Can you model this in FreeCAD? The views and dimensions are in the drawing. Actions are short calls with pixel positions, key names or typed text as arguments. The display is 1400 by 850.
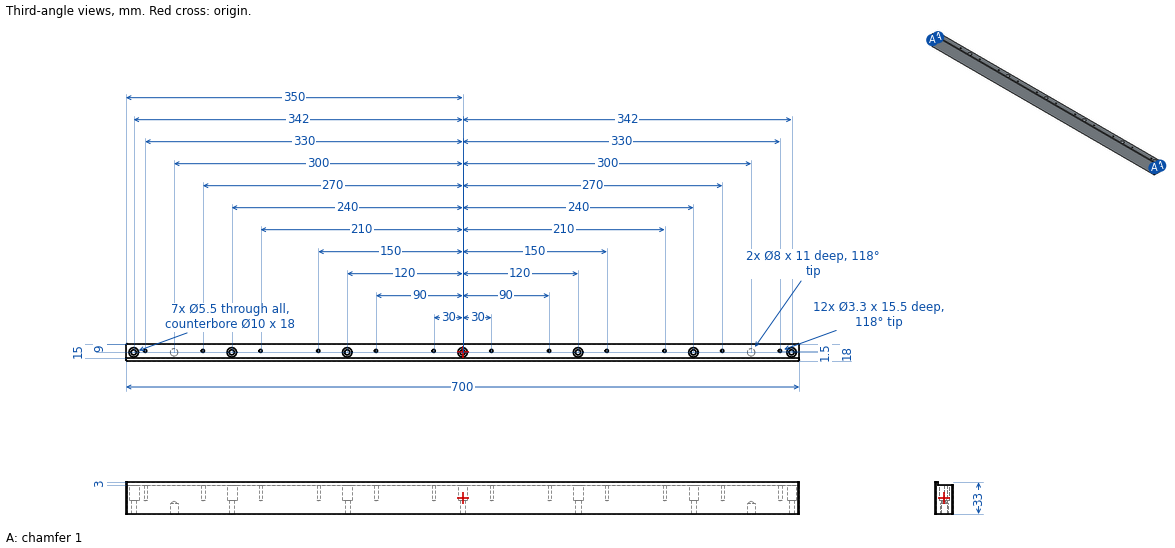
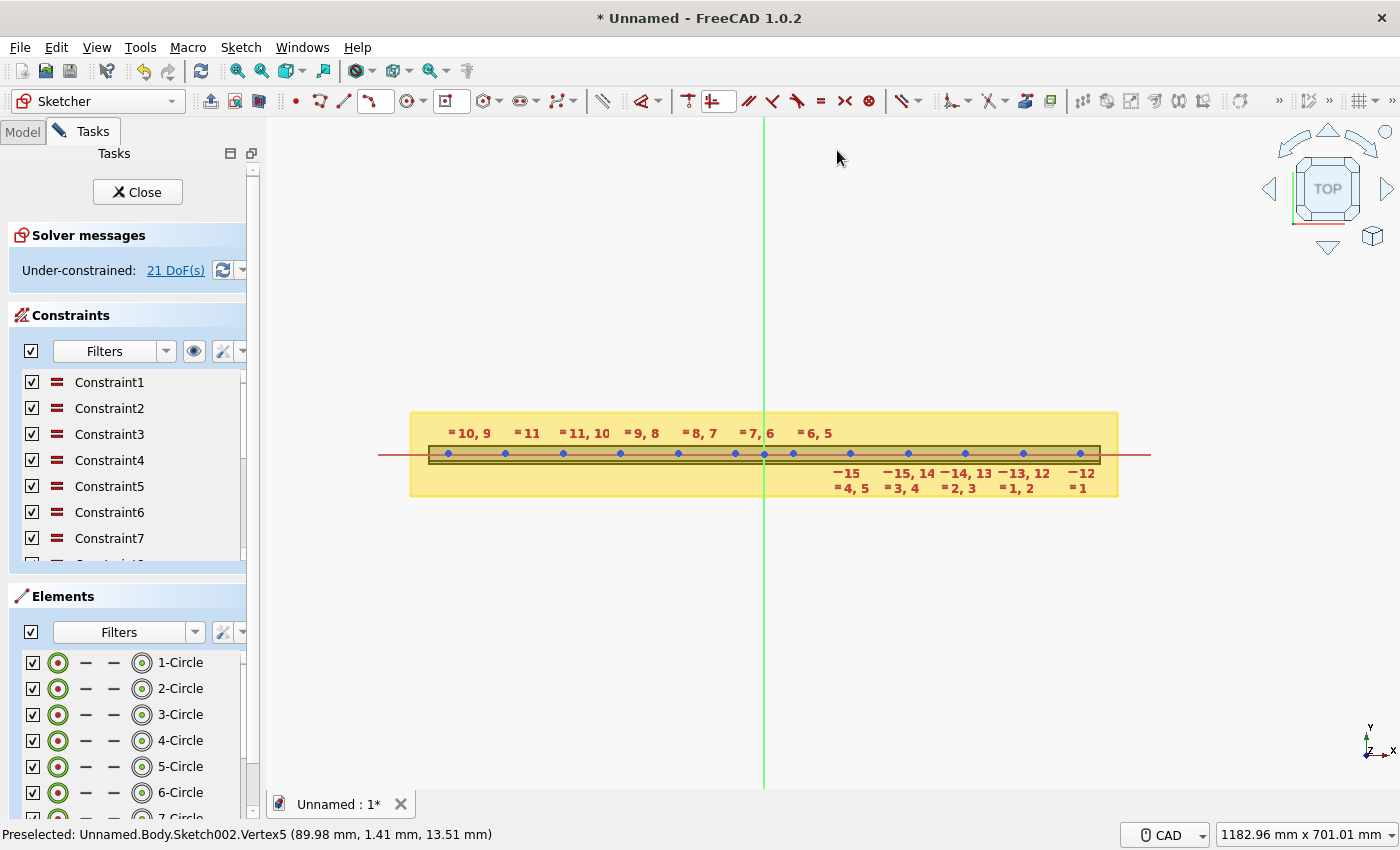
click(851, 453)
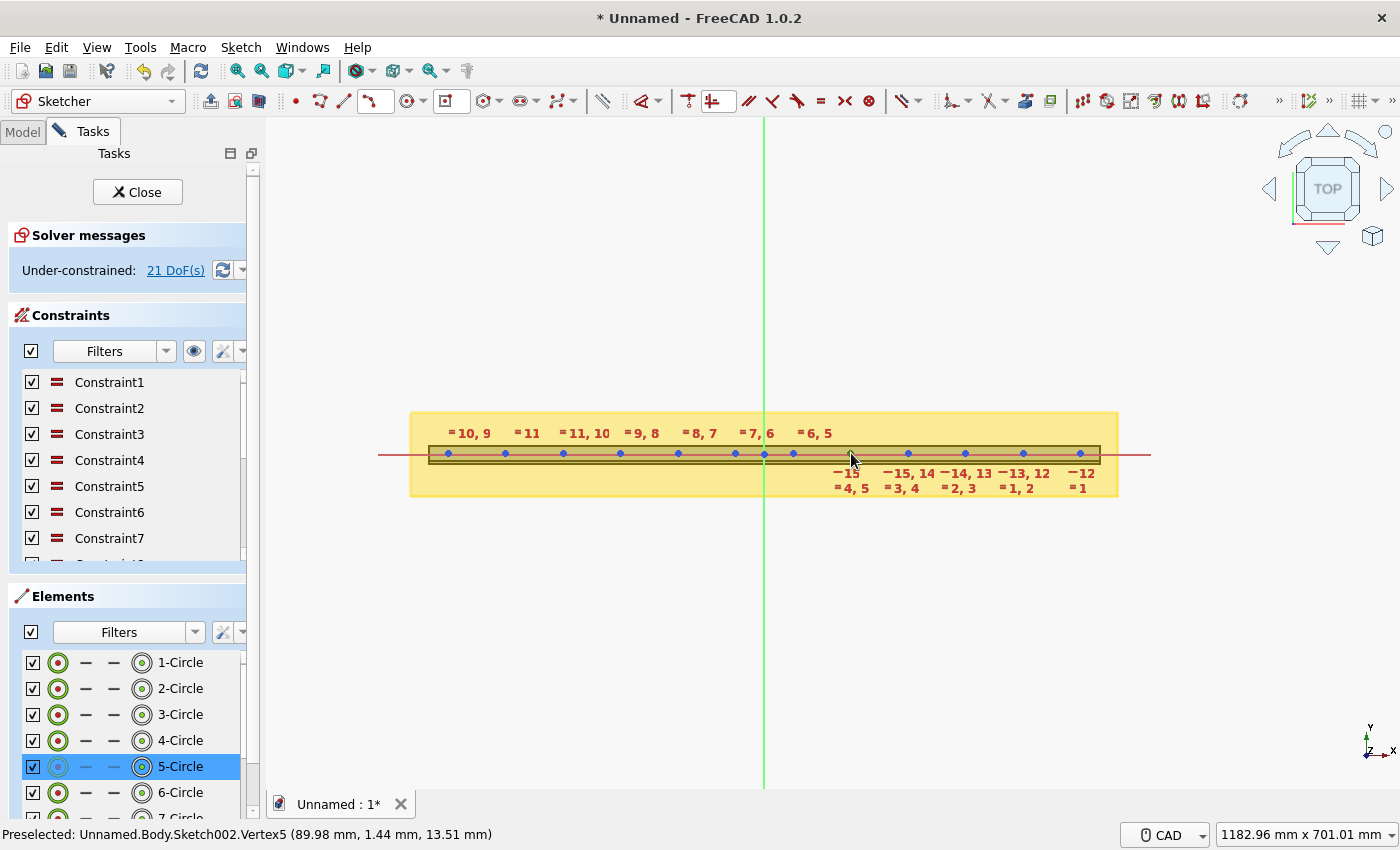
click(793, 454)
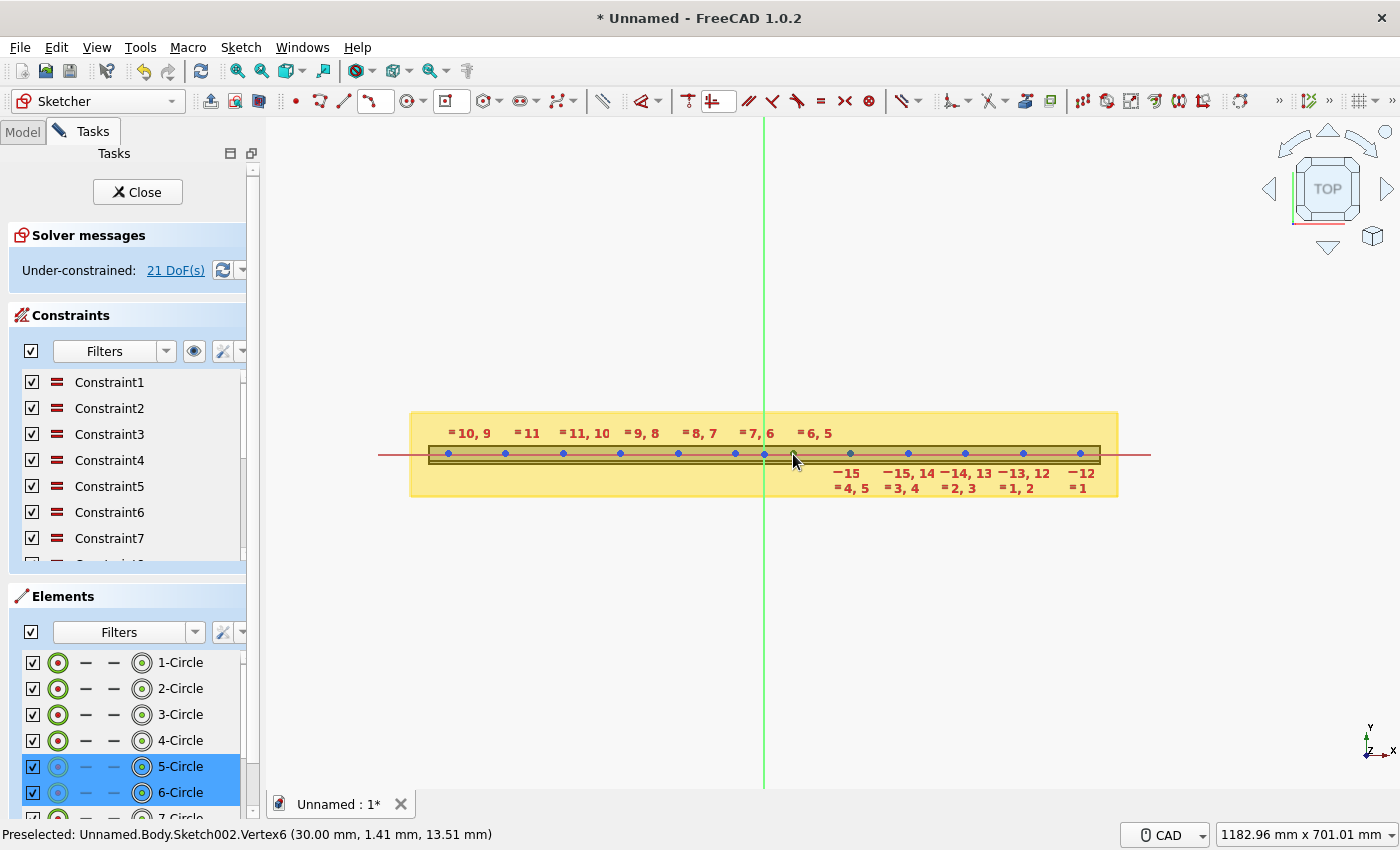
key(h)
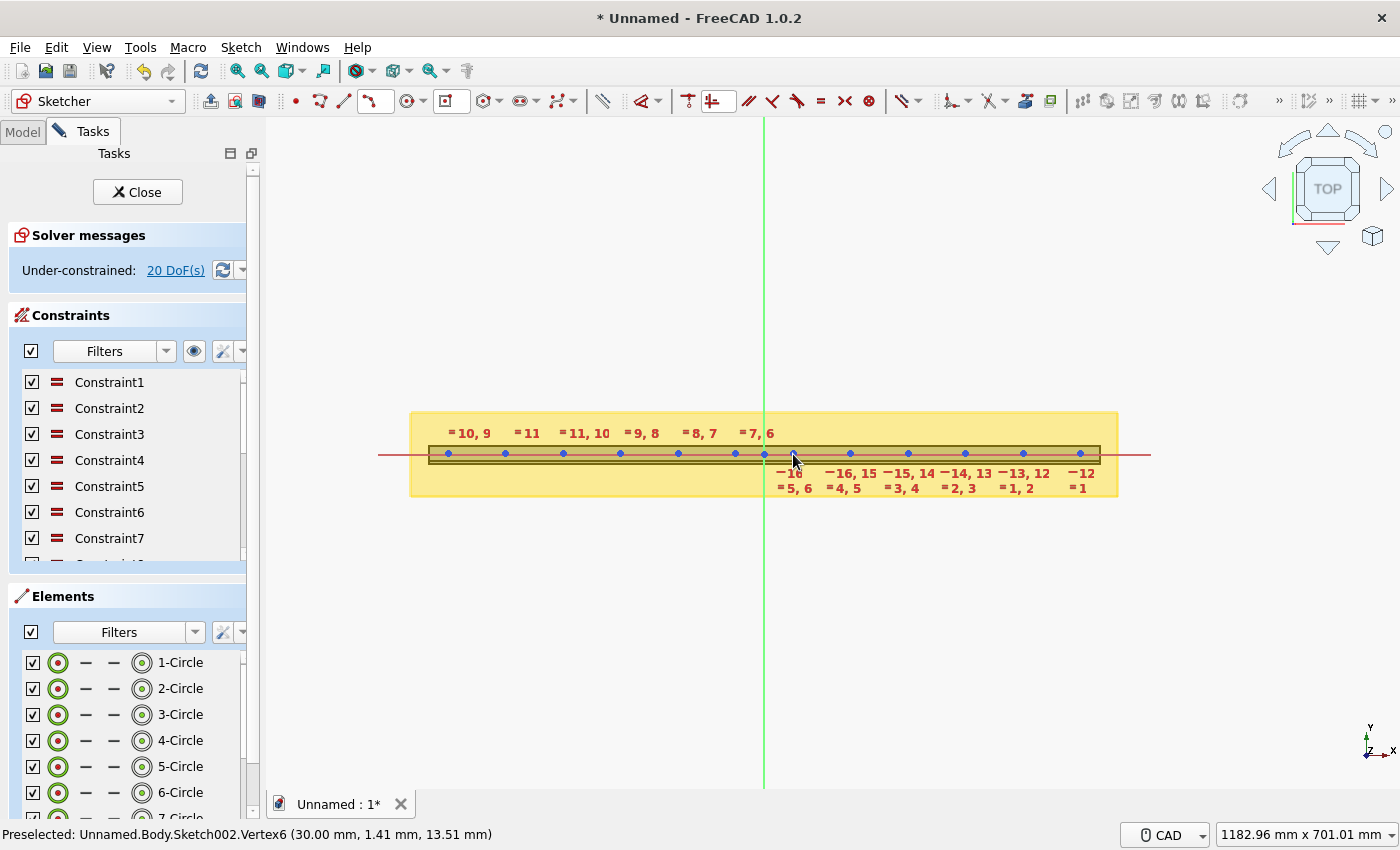
click(793, 453)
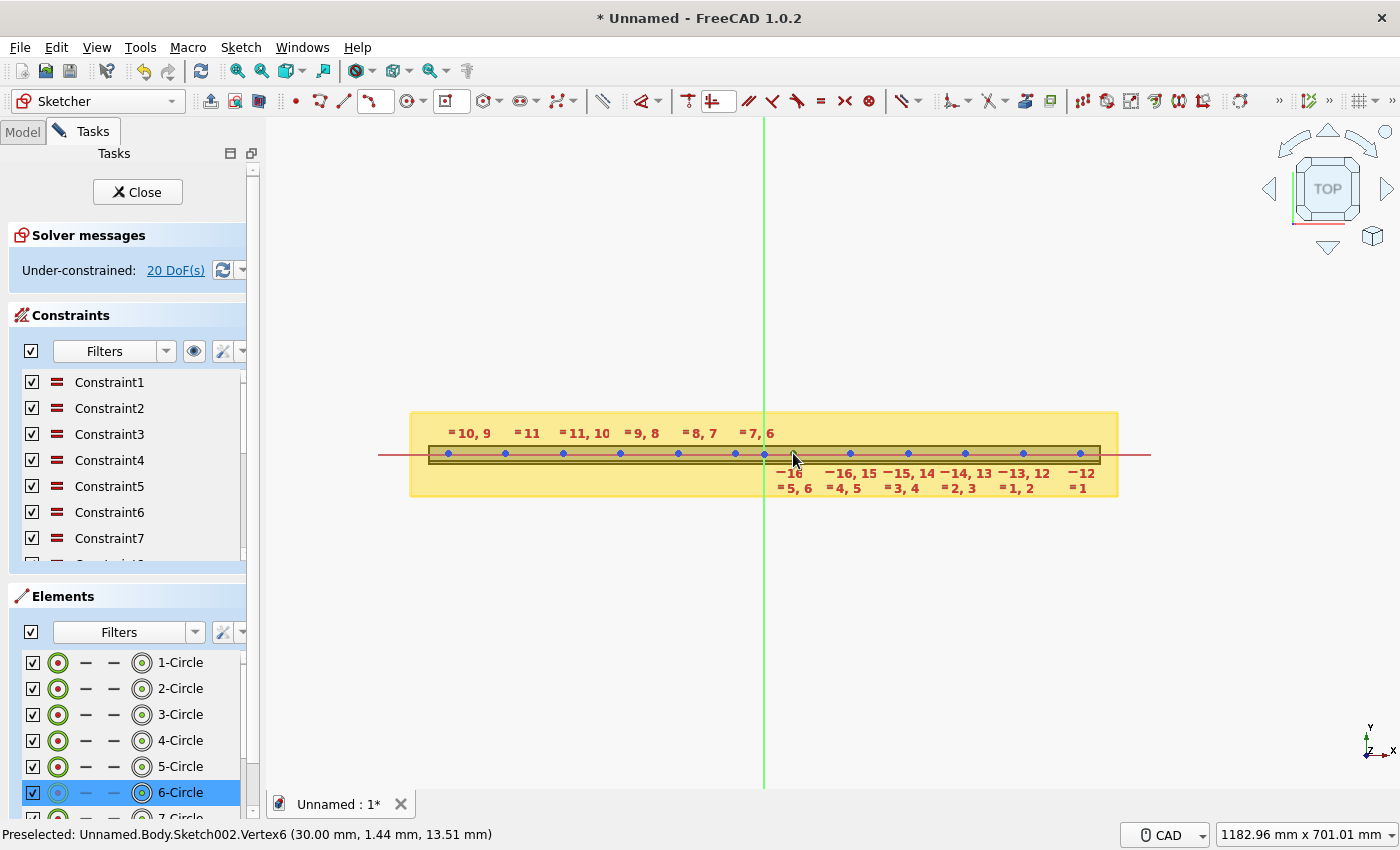
click(736, 454)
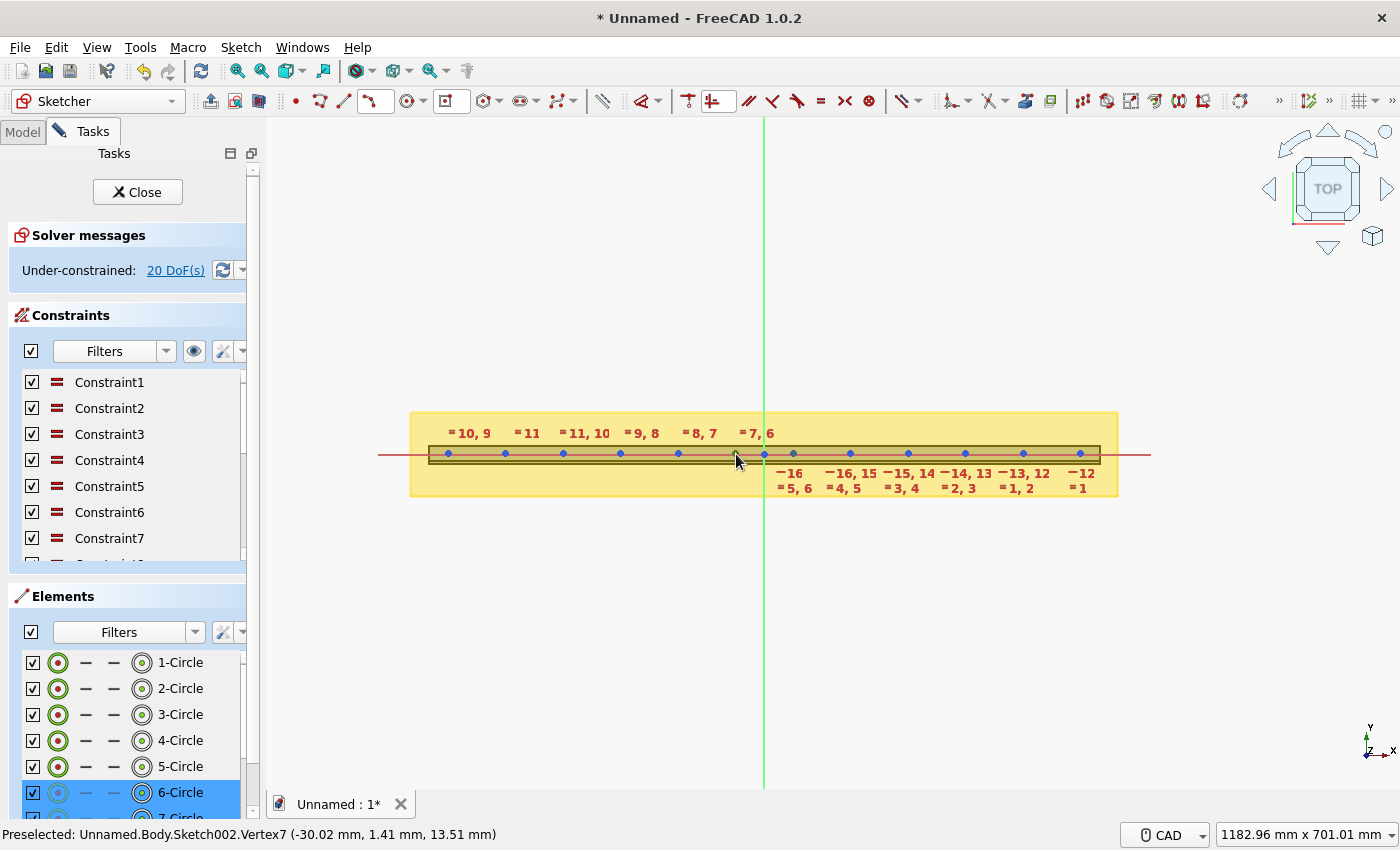
key(h)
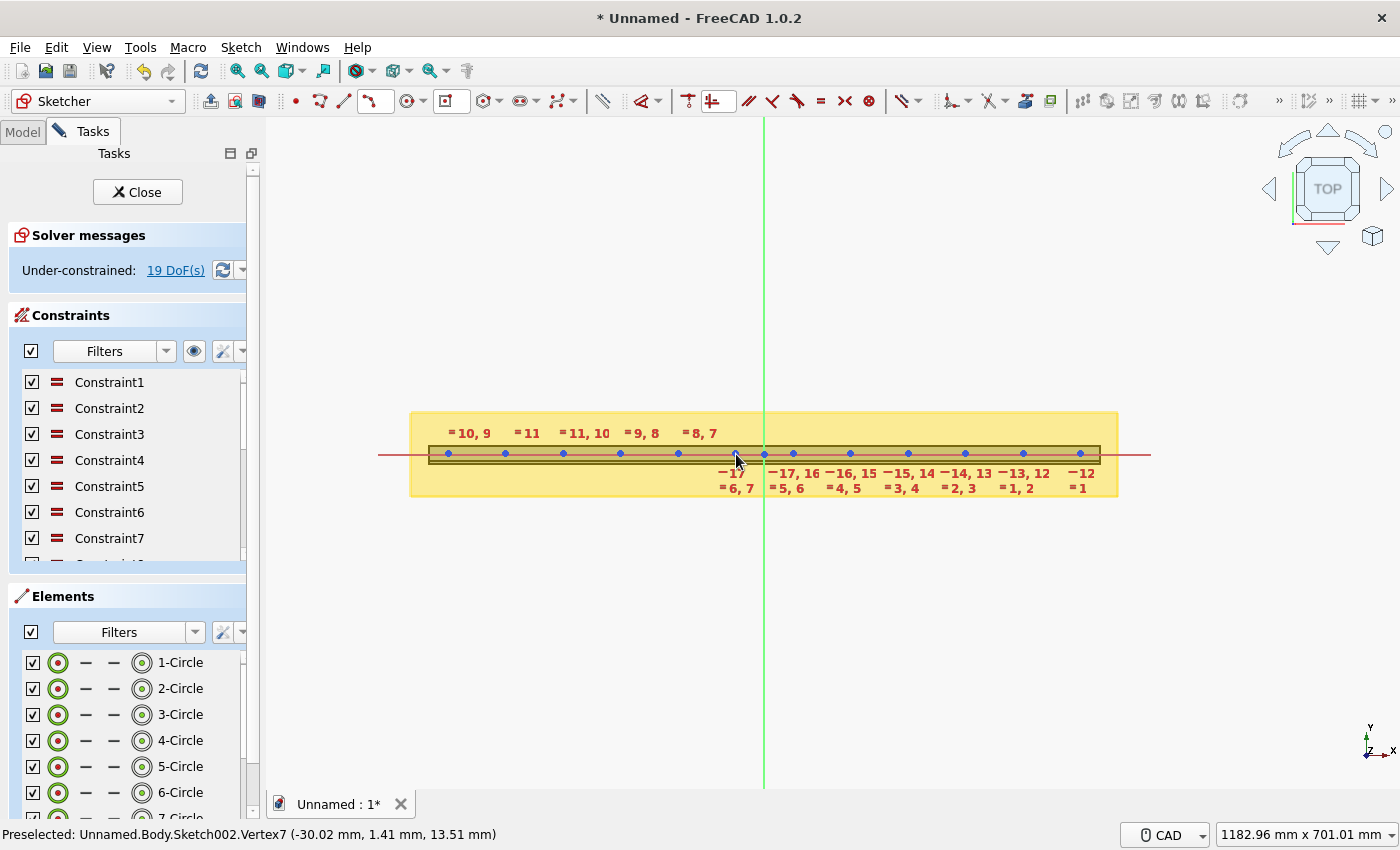
click(736, 453)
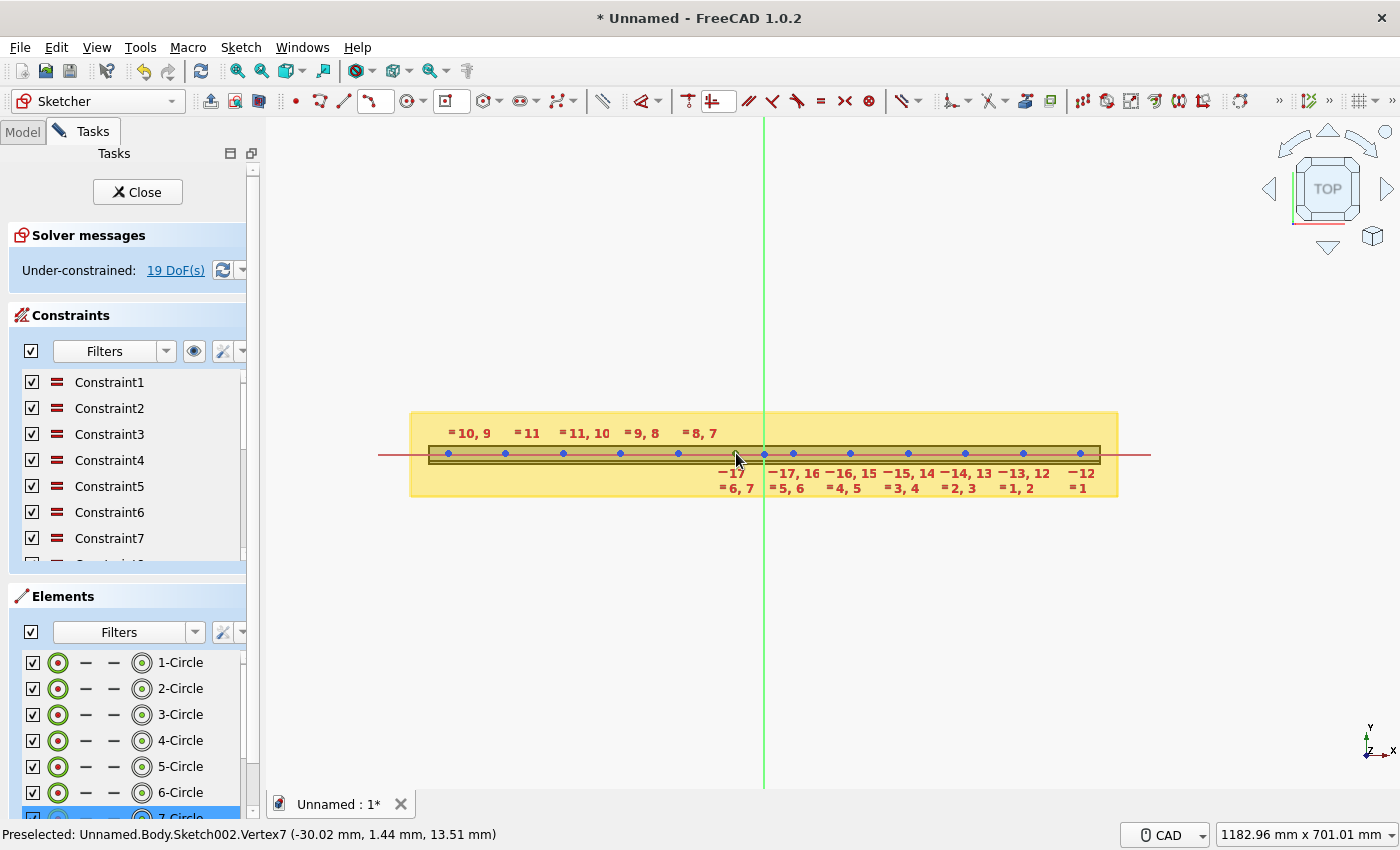
click(678, 454)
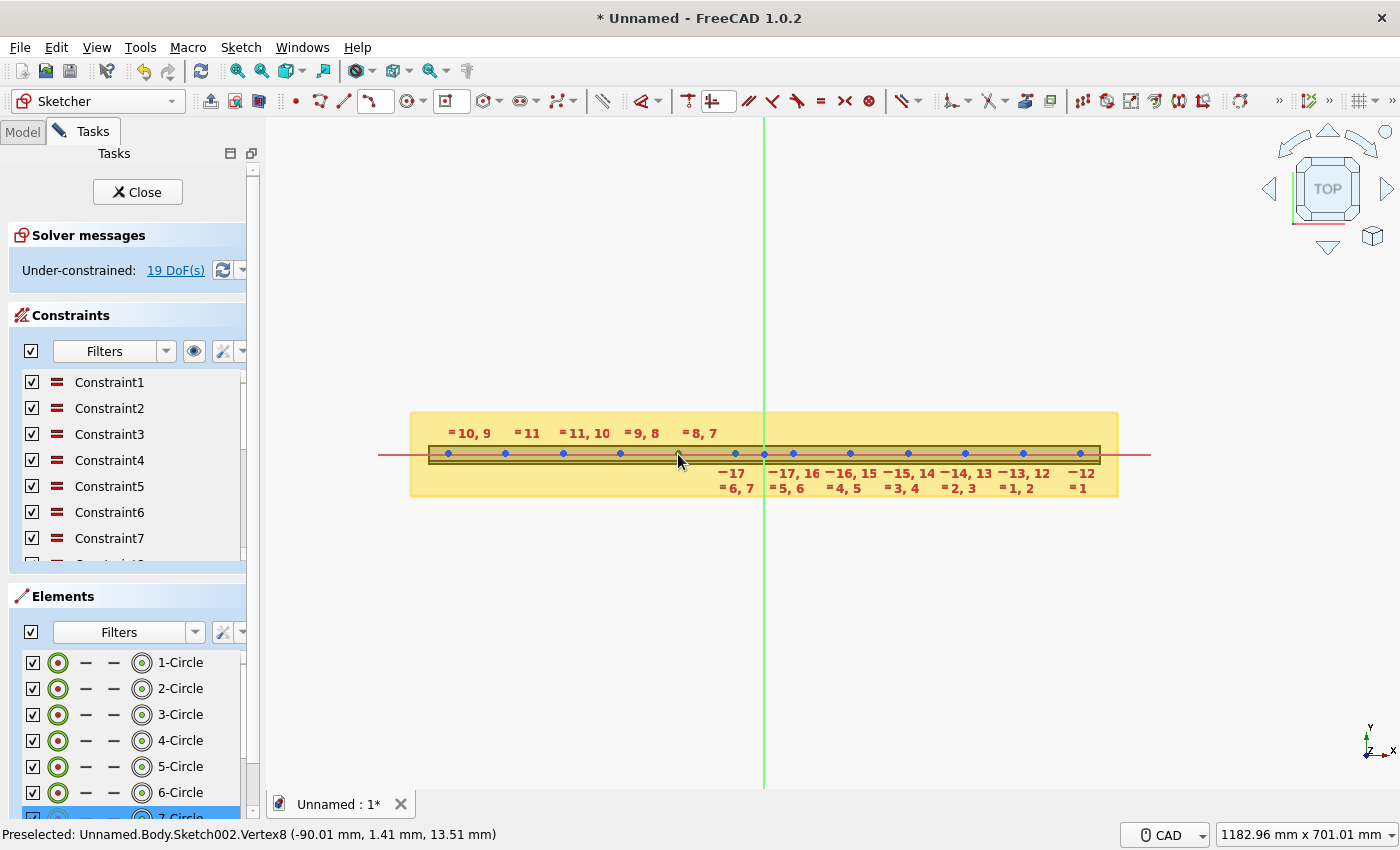
key(h)